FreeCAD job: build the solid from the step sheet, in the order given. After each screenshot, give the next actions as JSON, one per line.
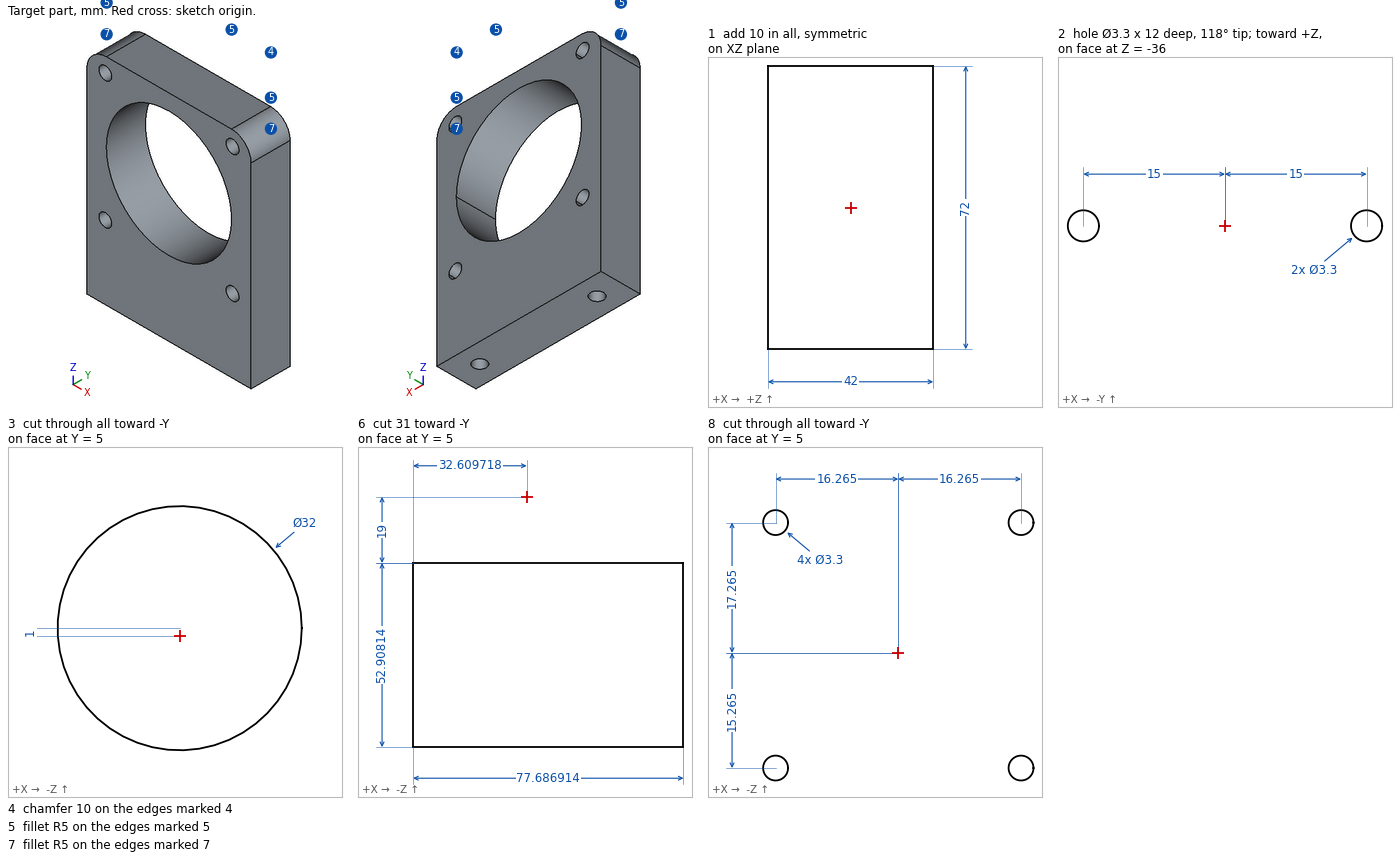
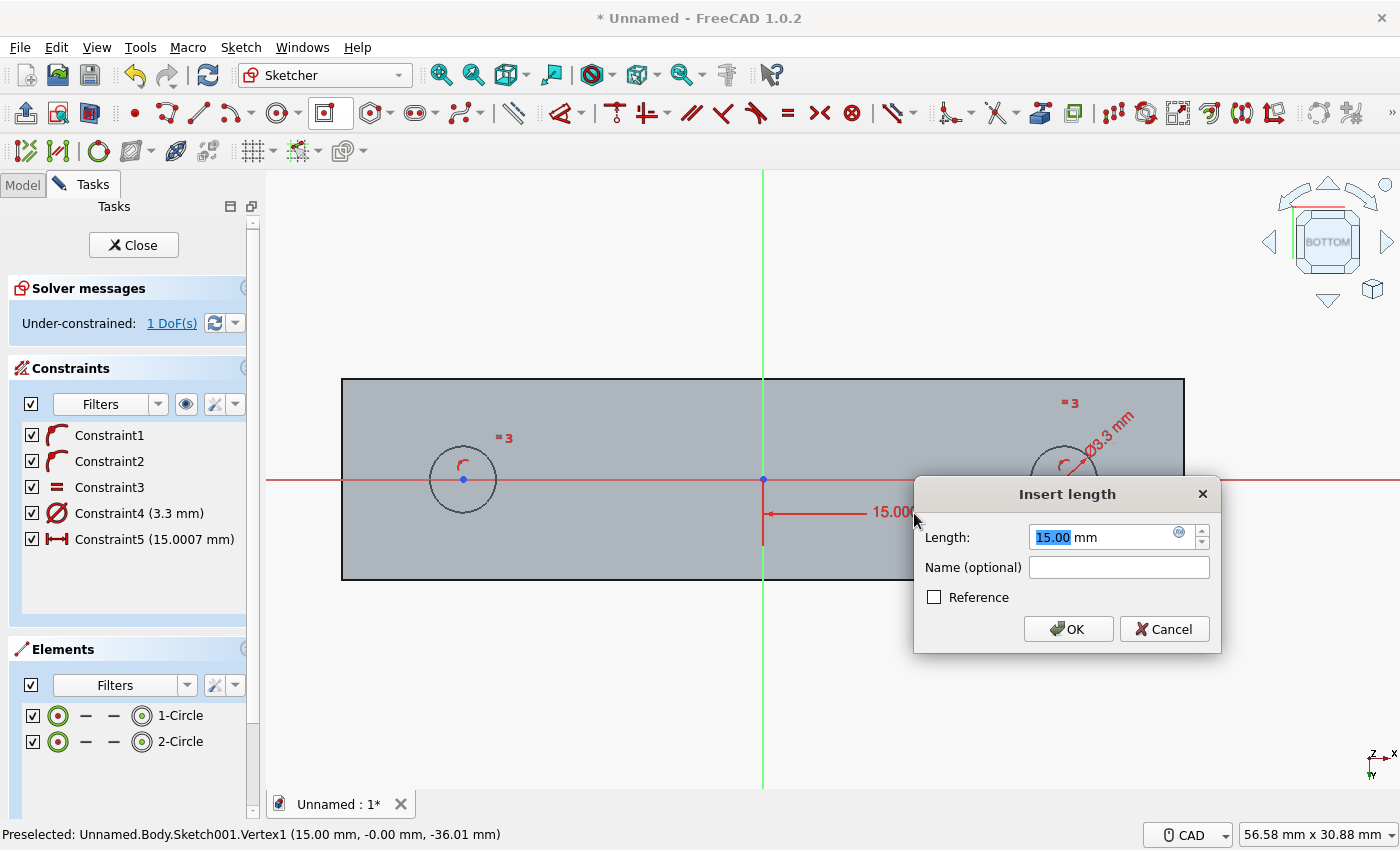
{"action": "type", "text": "15"}
{"action": "key", "text": "Return"}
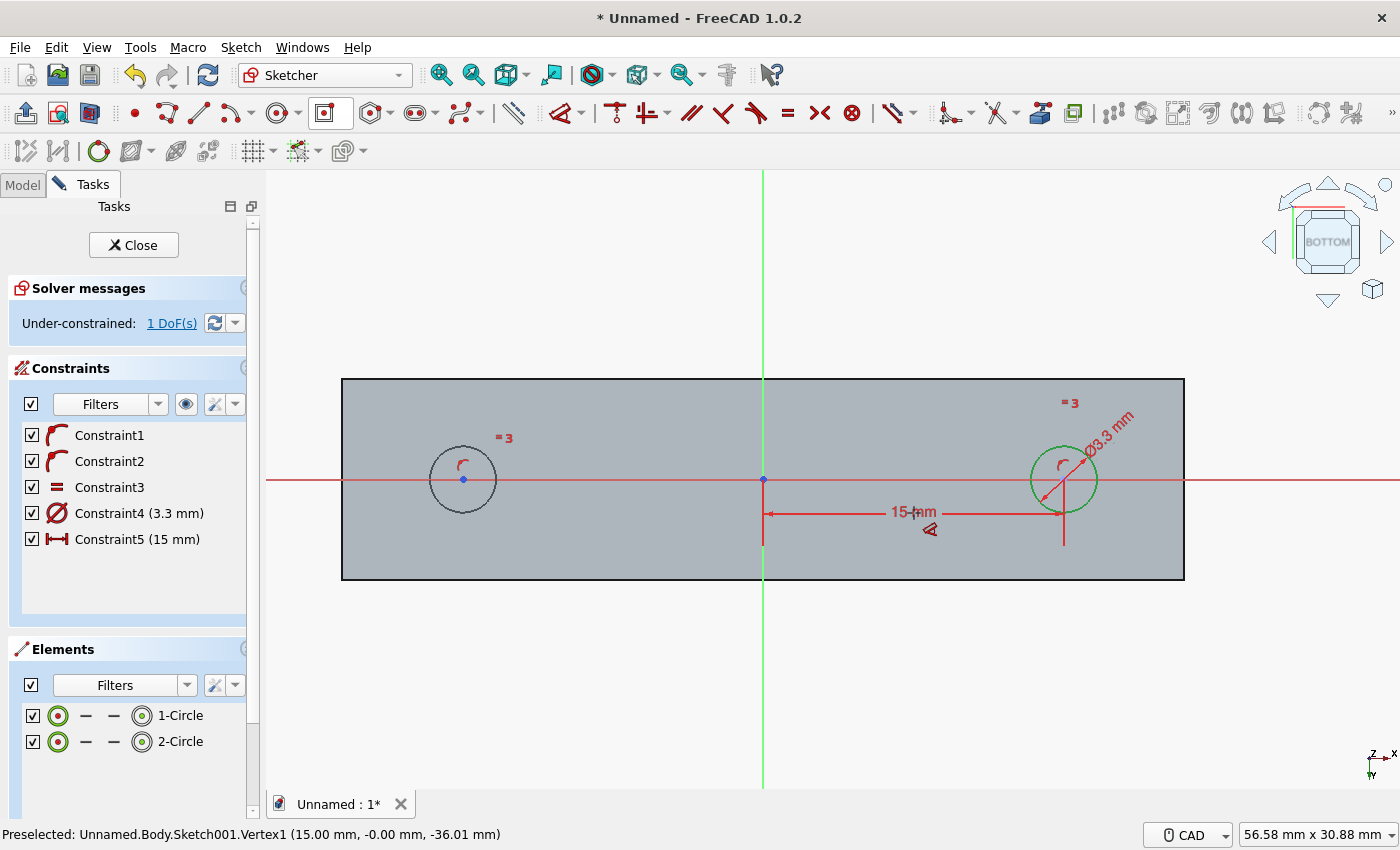
{"action": "left_click", "coordinate": [463, 479]}
{"action": "left_click", "coordinate": [613, 513]}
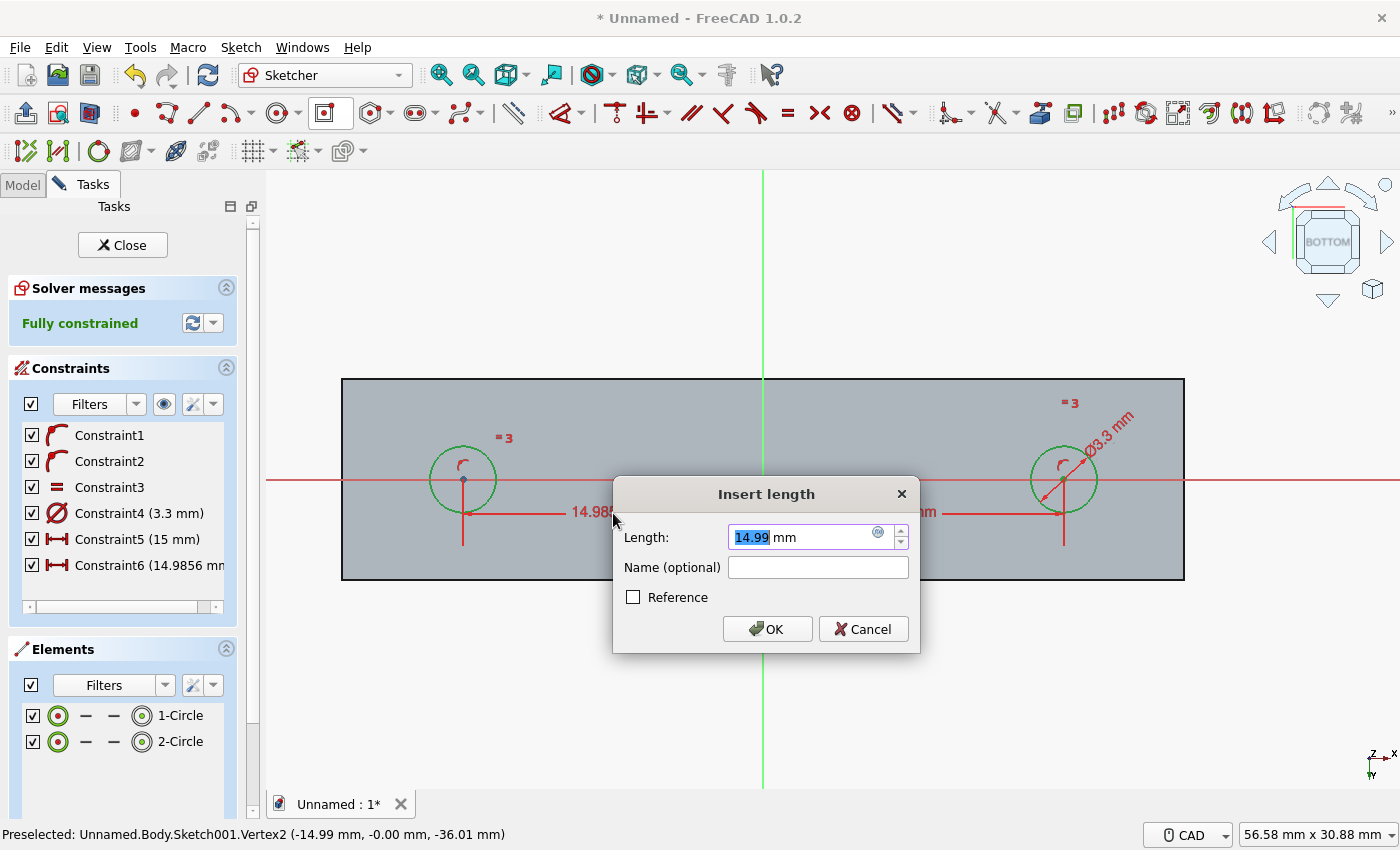
{"action": "type", "text": "15"}
{"action": "key", "text": "Return"}
{"action": "key", "text": "Escape"}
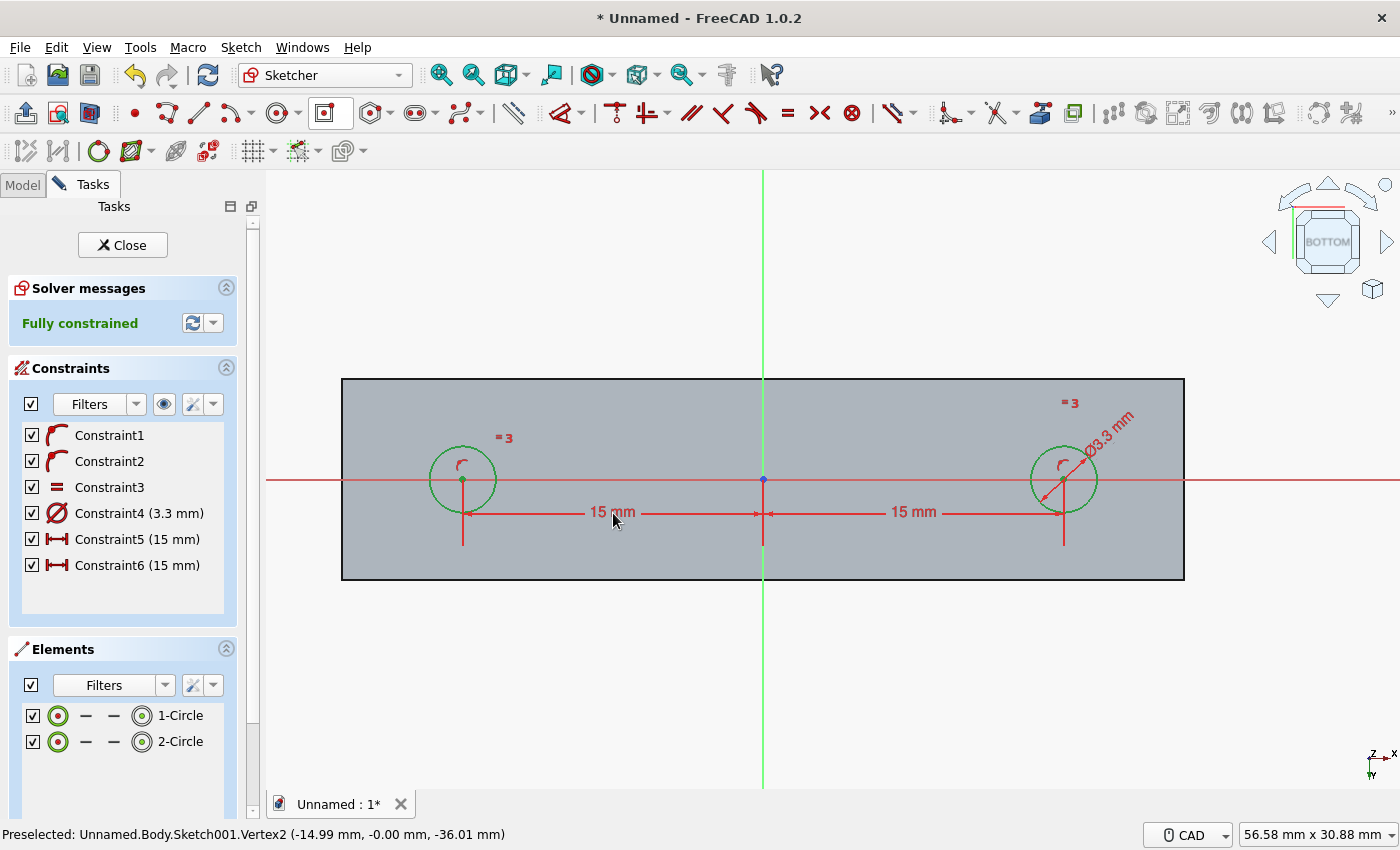
{"action": "left_click", "coordinate": [123, 245]}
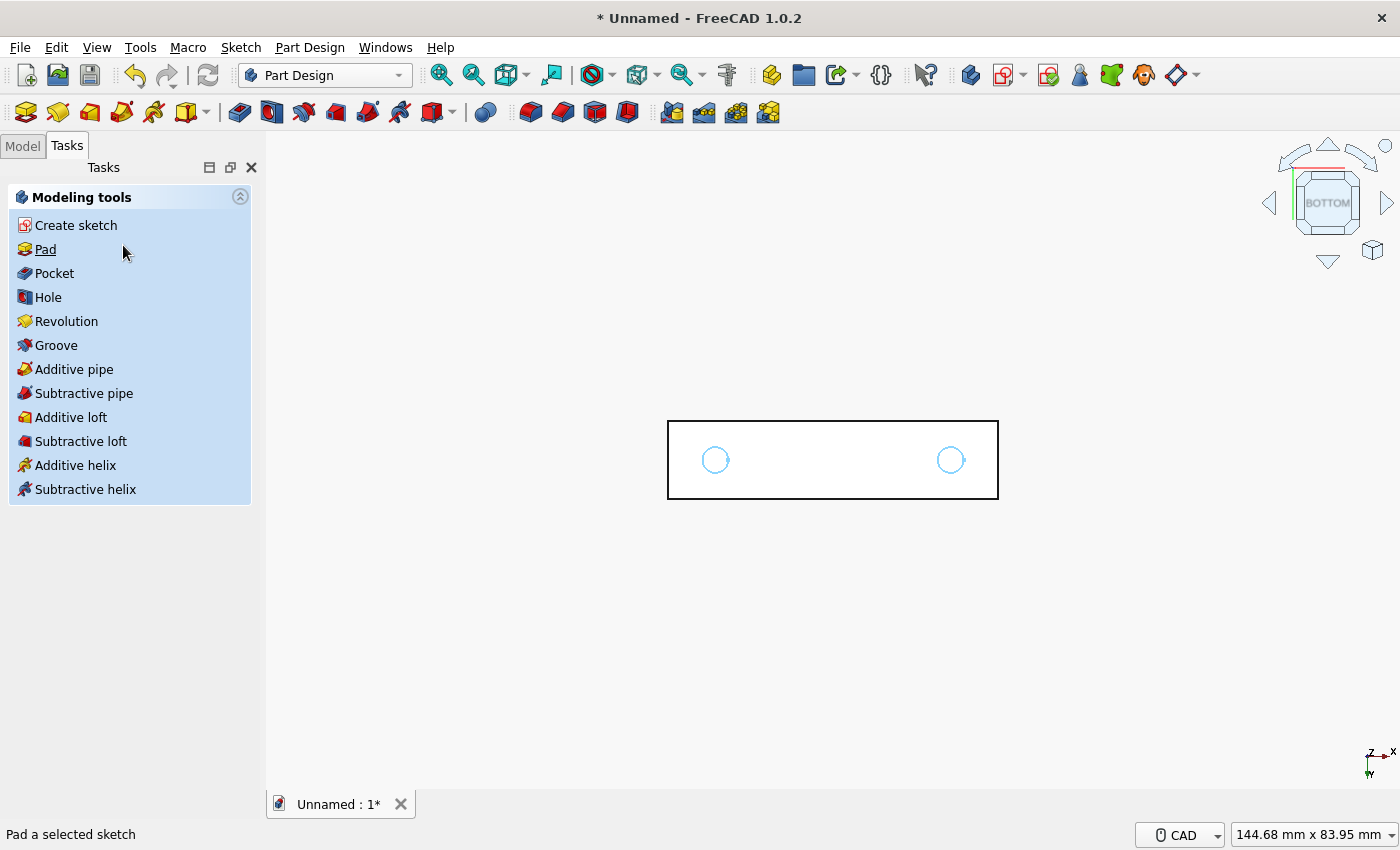
{"action": "left_click", "coordinate": [272, 112]}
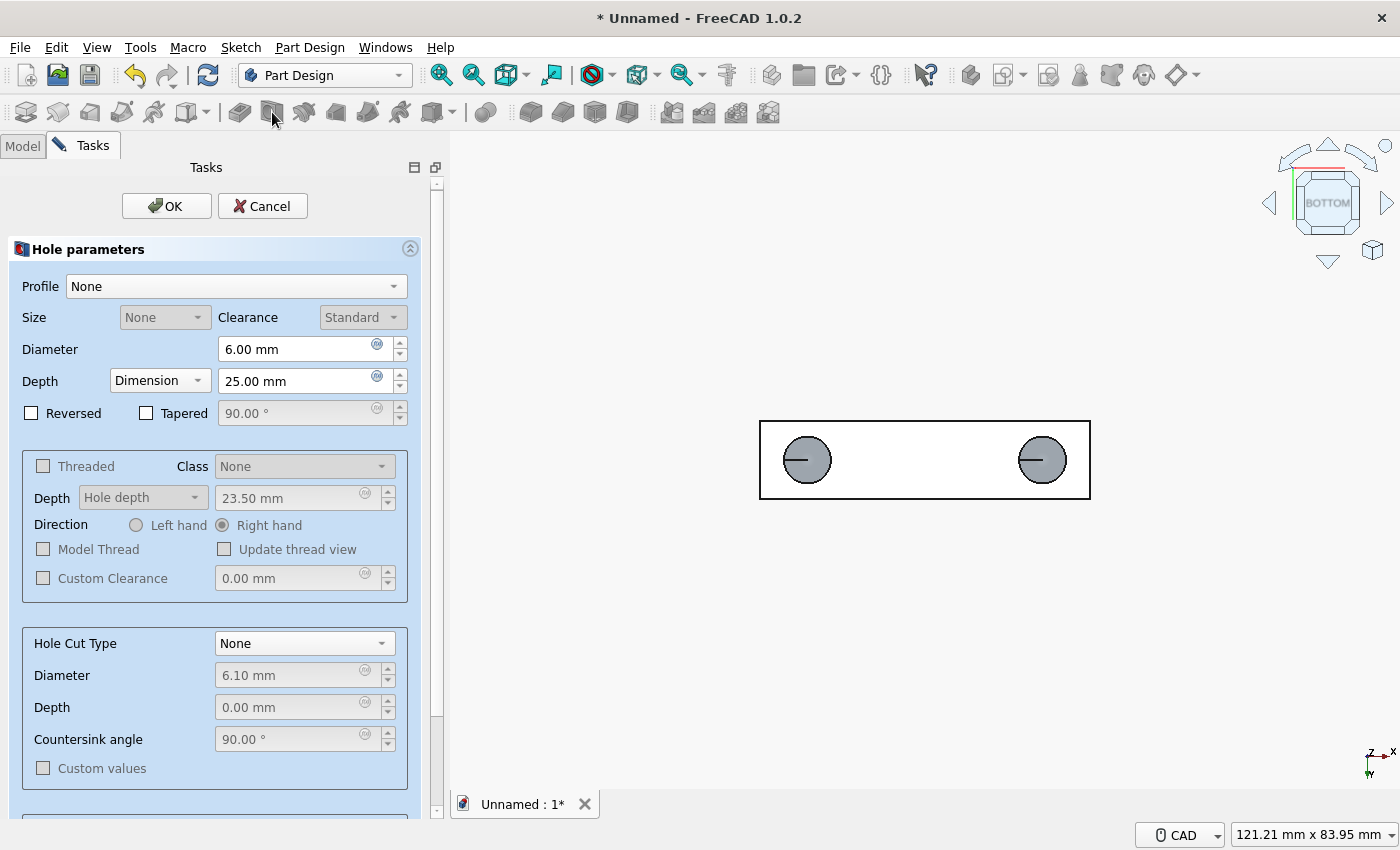
{"action": "triple_click", "coordinate": [305, 349]}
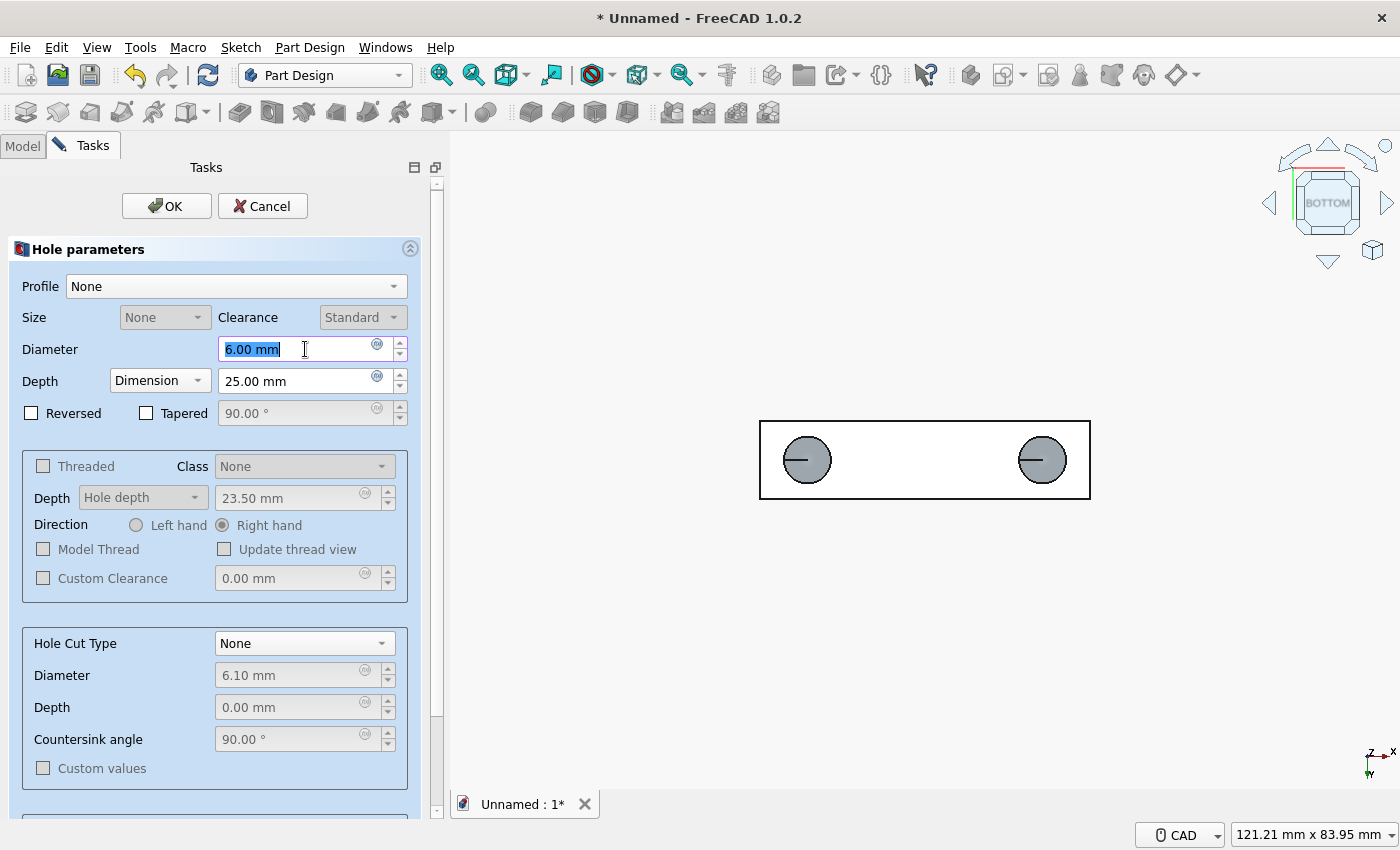
{"action": "type", "text": "3.3"}
{"action": "key", "text": "Tab"}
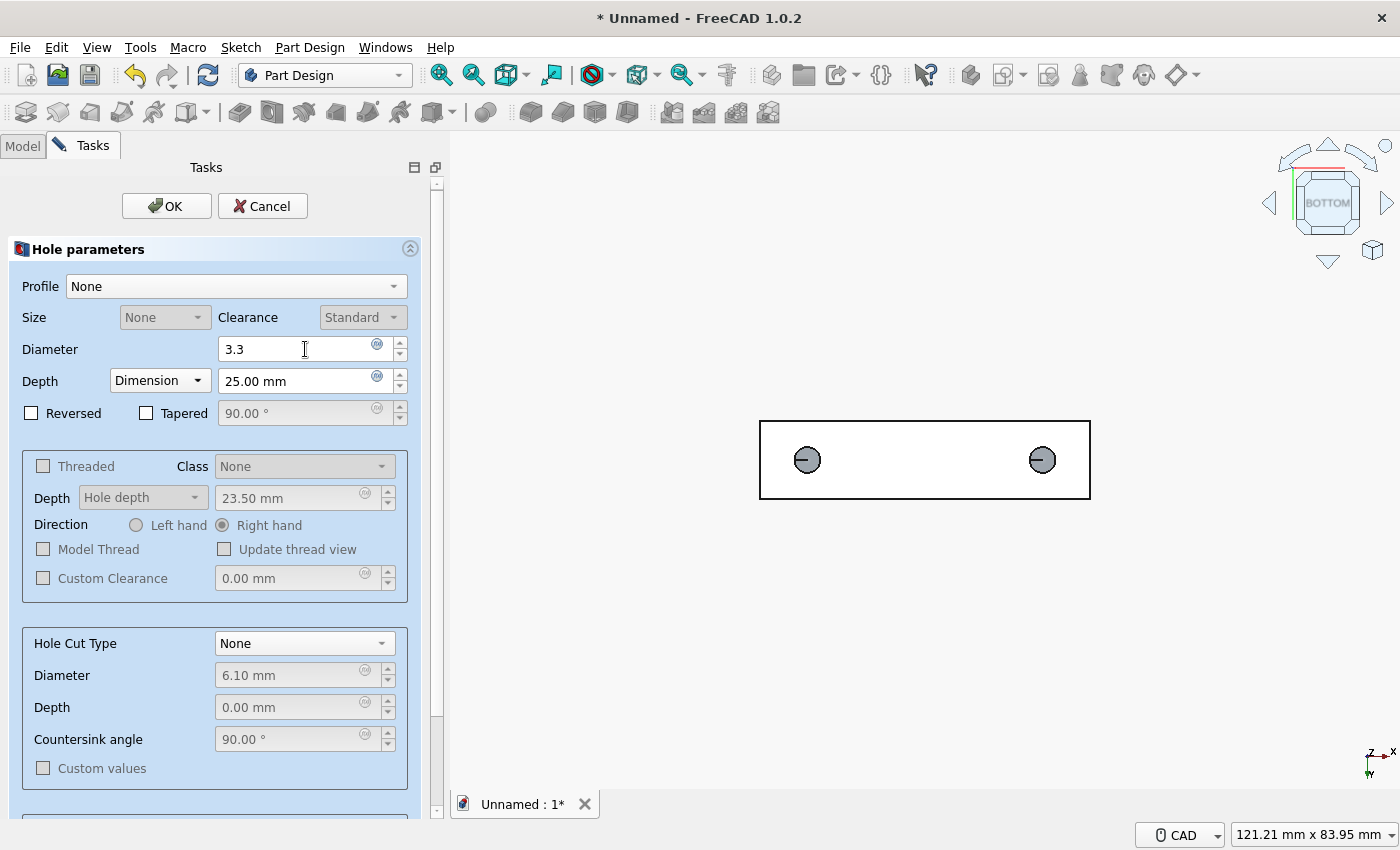
{"action": "triple_click", "coordinate": [305, 381]}